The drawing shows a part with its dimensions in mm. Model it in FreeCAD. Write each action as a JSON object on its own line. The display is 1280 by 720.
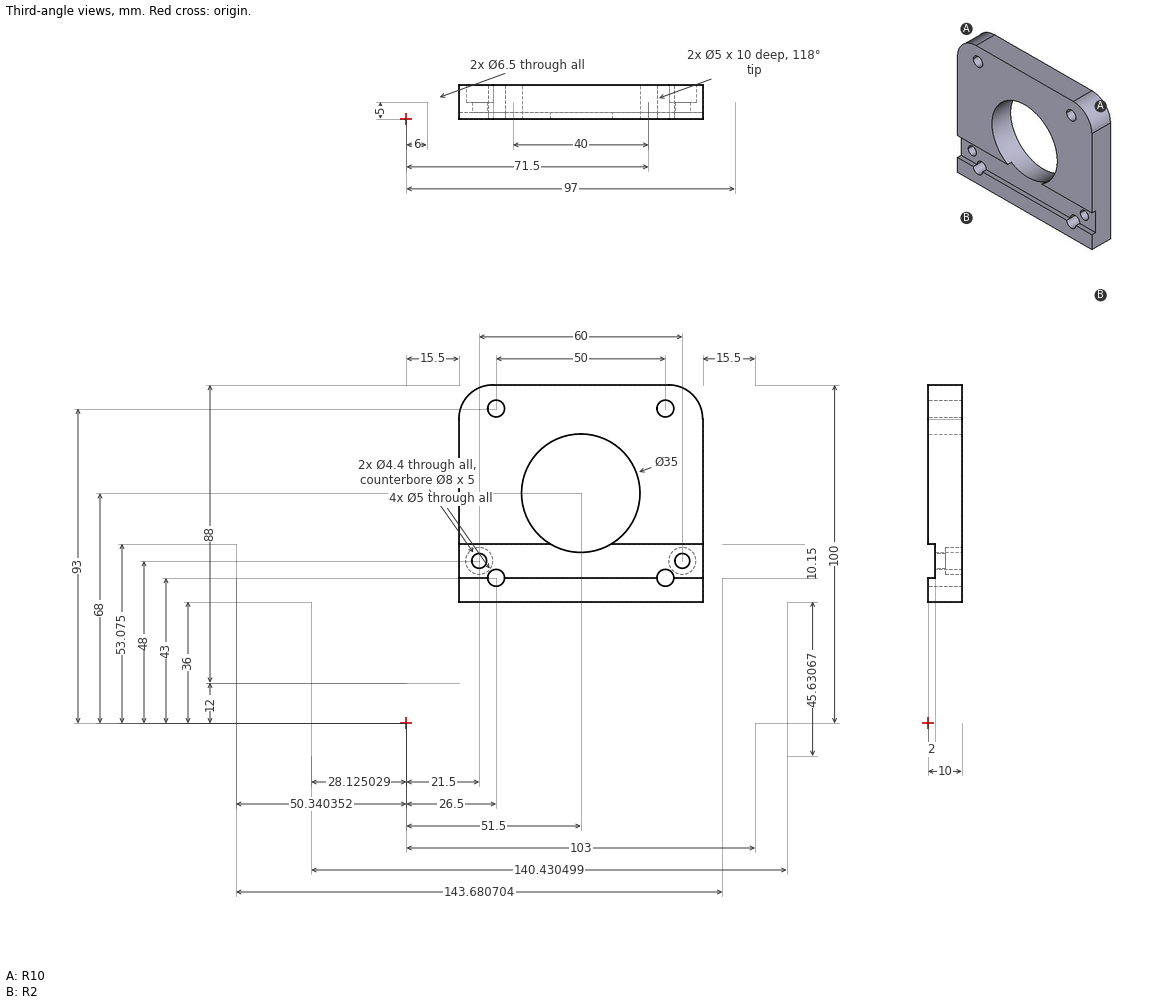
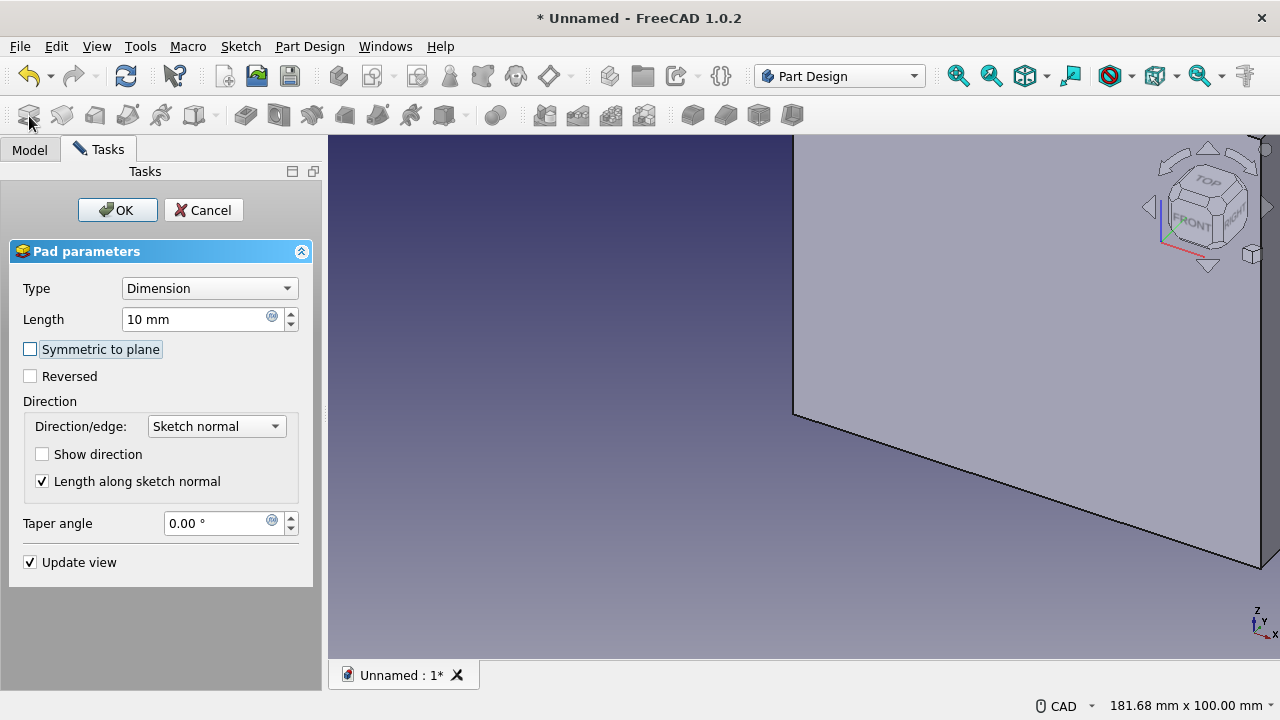
{"action": "left_click", "coordinate": [31, 376]}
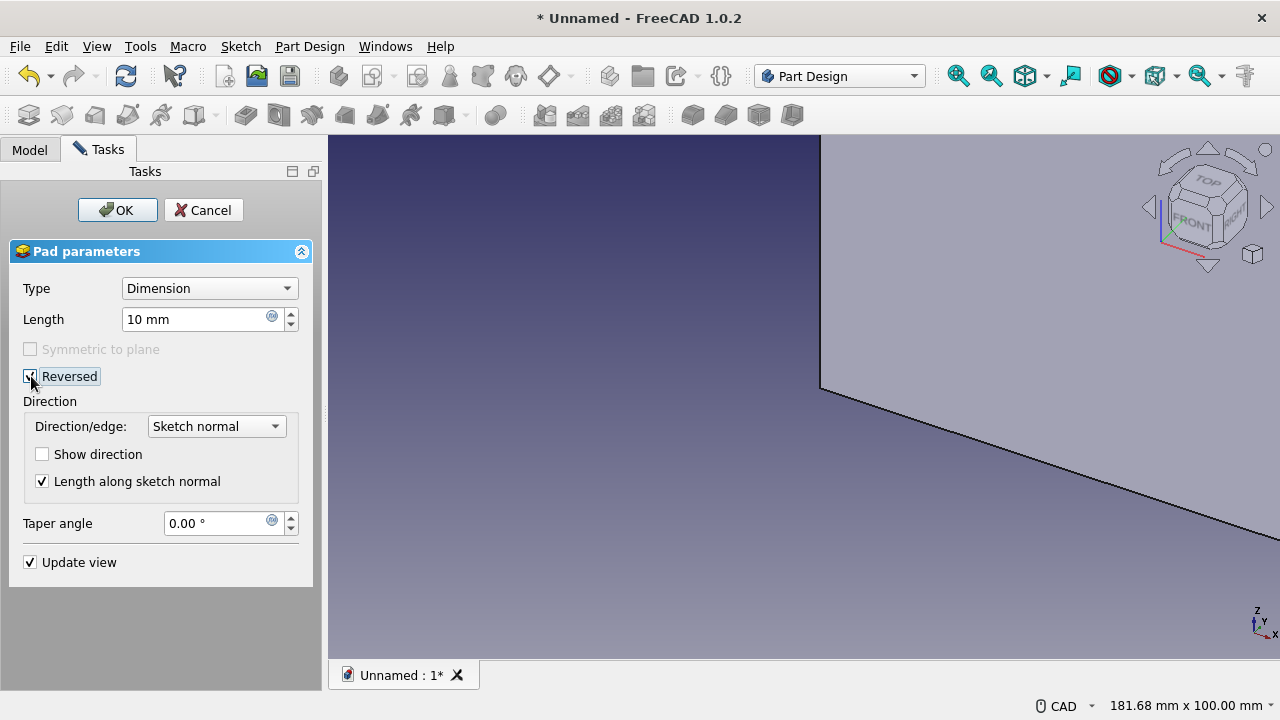
{"action": "left_click", "coordinate": [118, 210]}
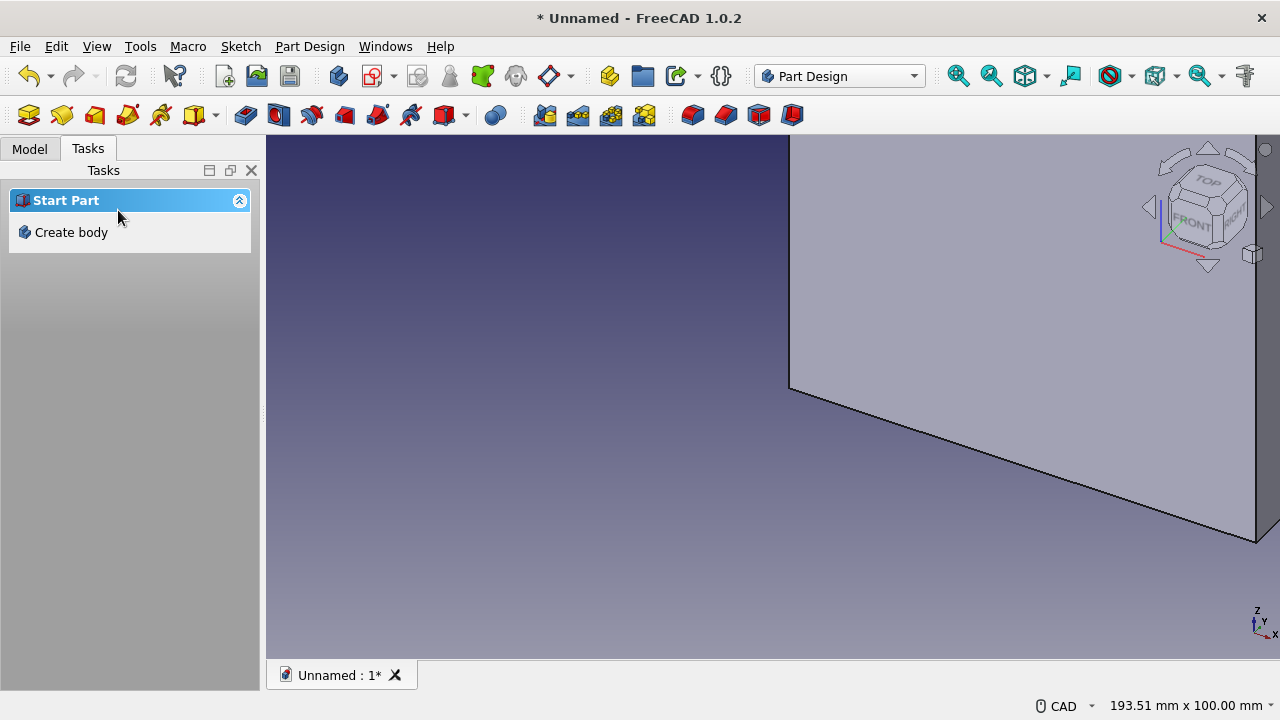
{"action": "left_click", "coordinate": [959, 76]}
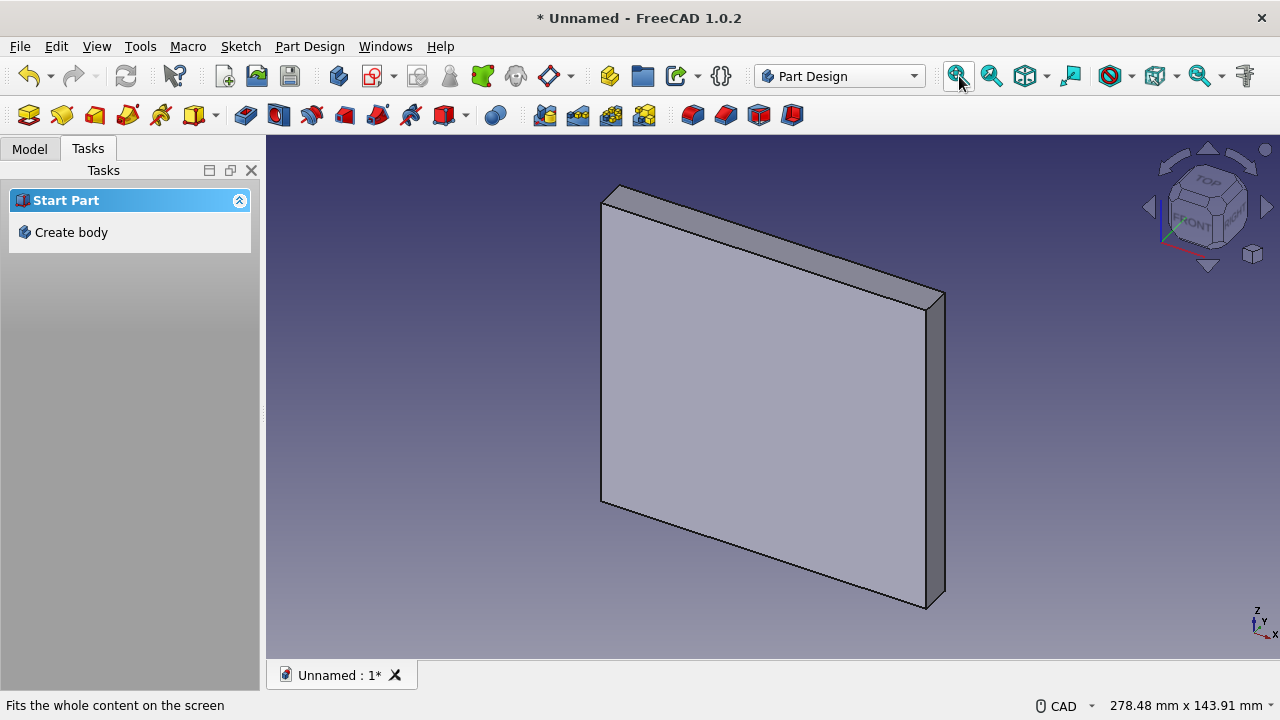
{"action": "key", "text": "4"}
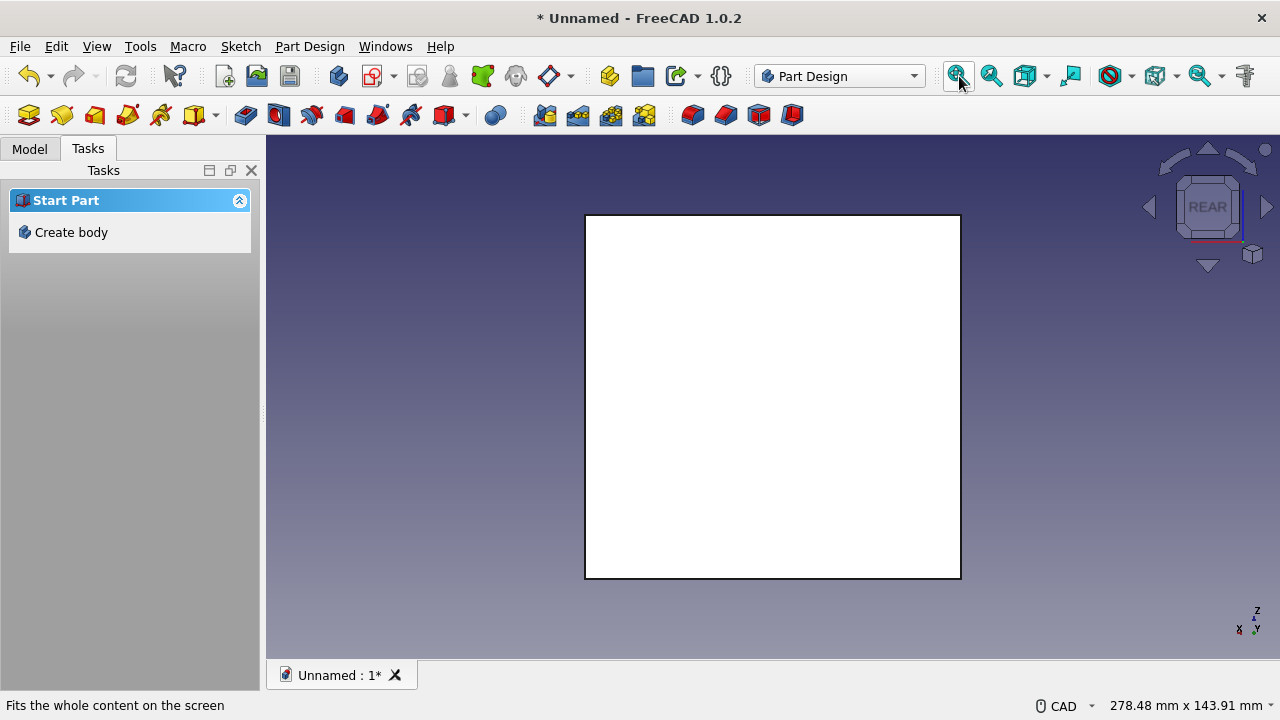
{"action": "left_click", "coordinate": [773, 396]}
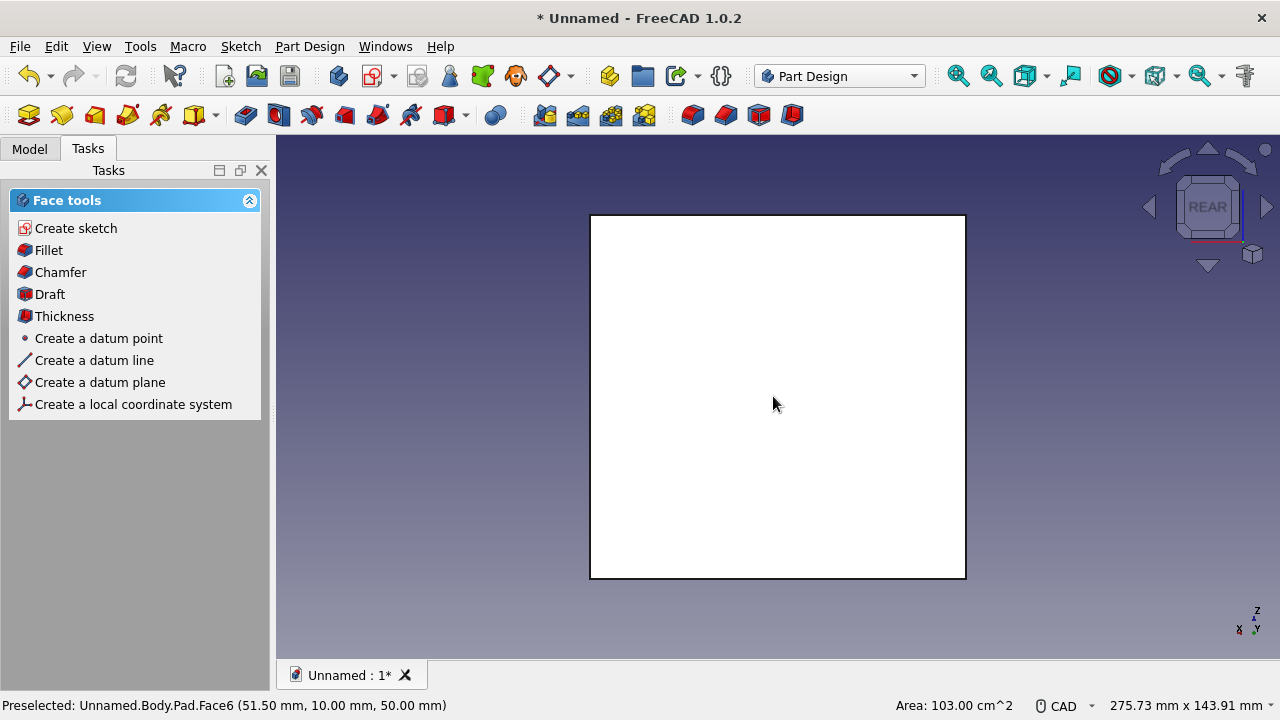
{"action": "left_click", "coordinate": [372, 76]}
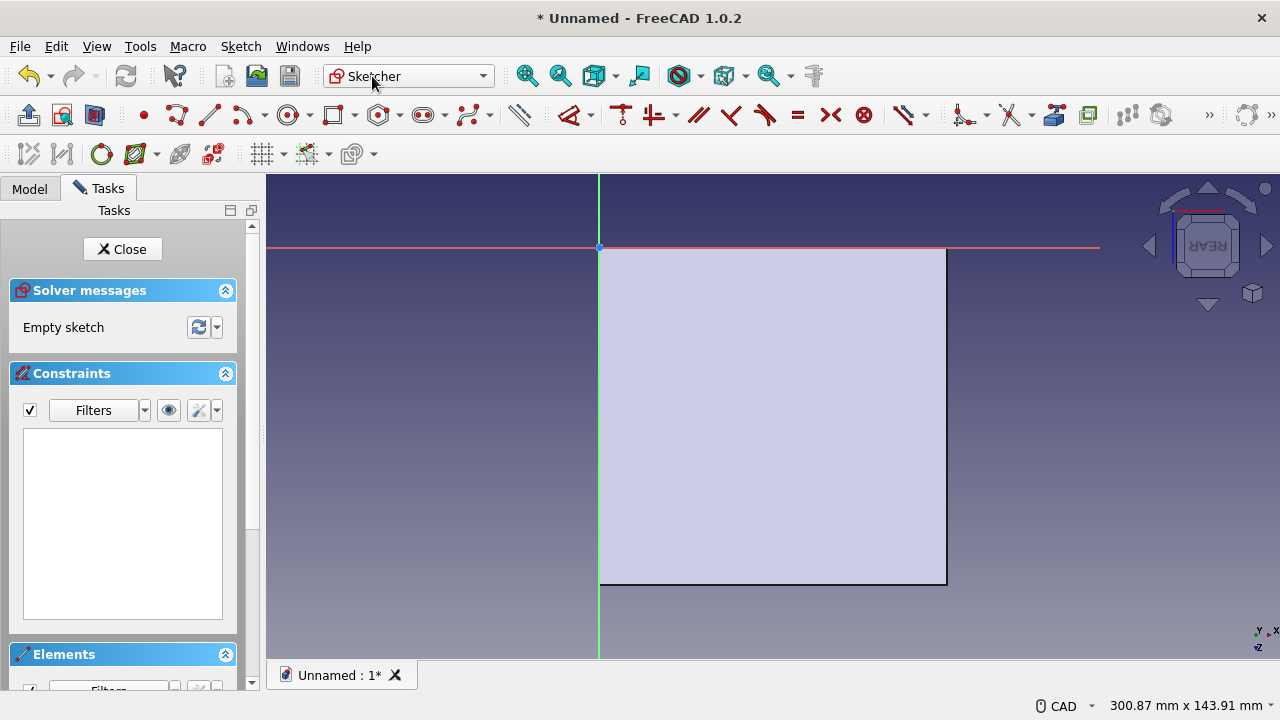
{"action": "left_click", "coordinate": [332, 116]}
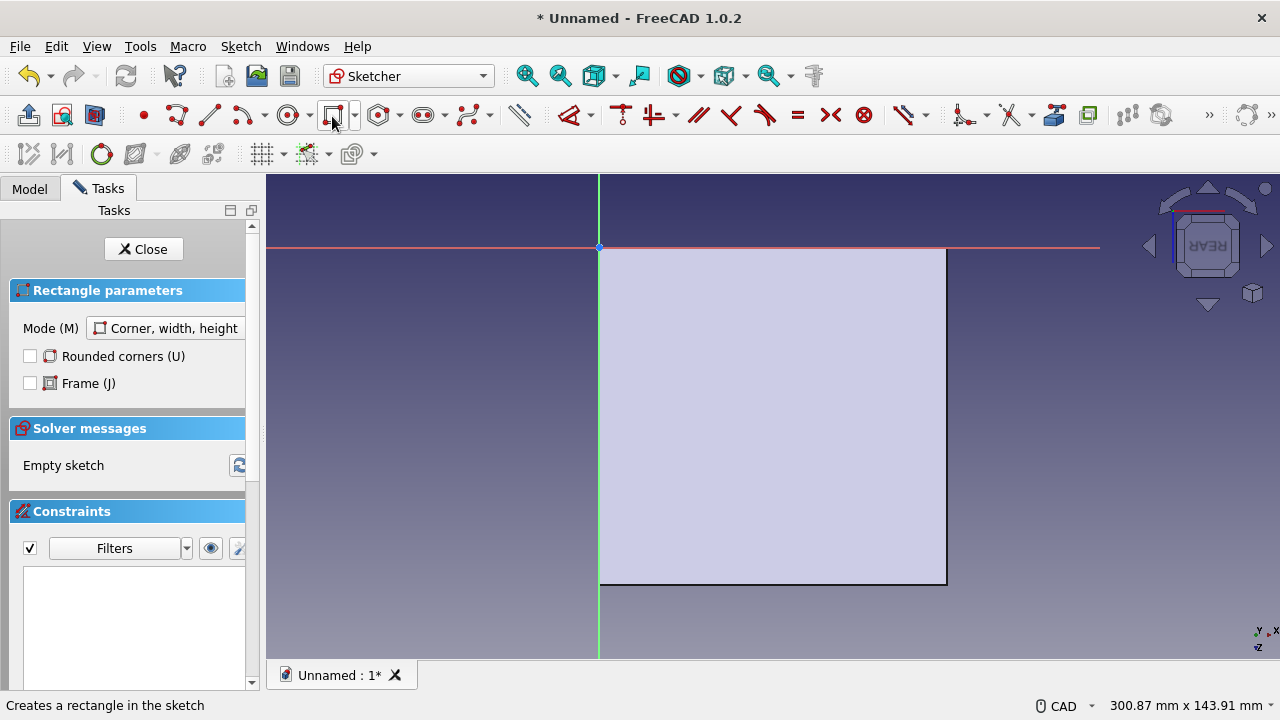
{"action": "left_click", "coordinate": [599, 288]}
{"action": "mouse_move", "coordinate": [652, 585]}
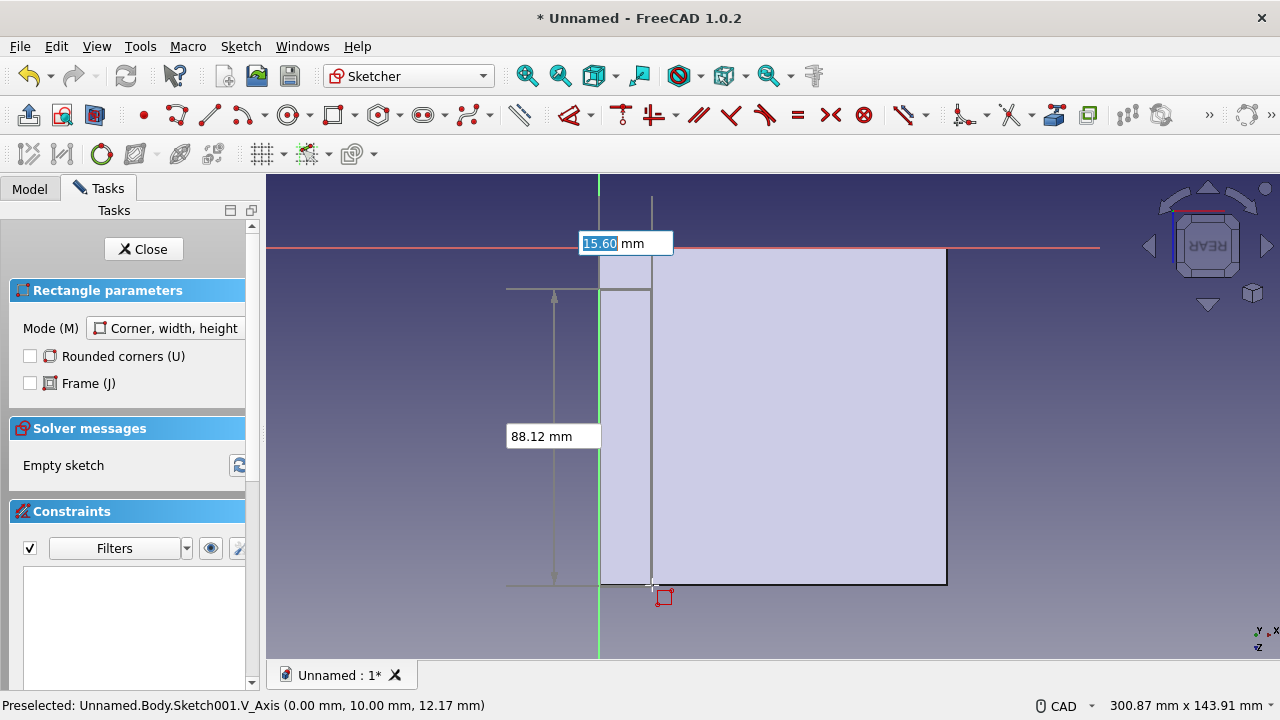
{"action": "type", "text": "15.5"}
{"action": "key", "text": "Tab"}
{"action": "type", "text": "88"}
{"action": "key", "text": "Return"}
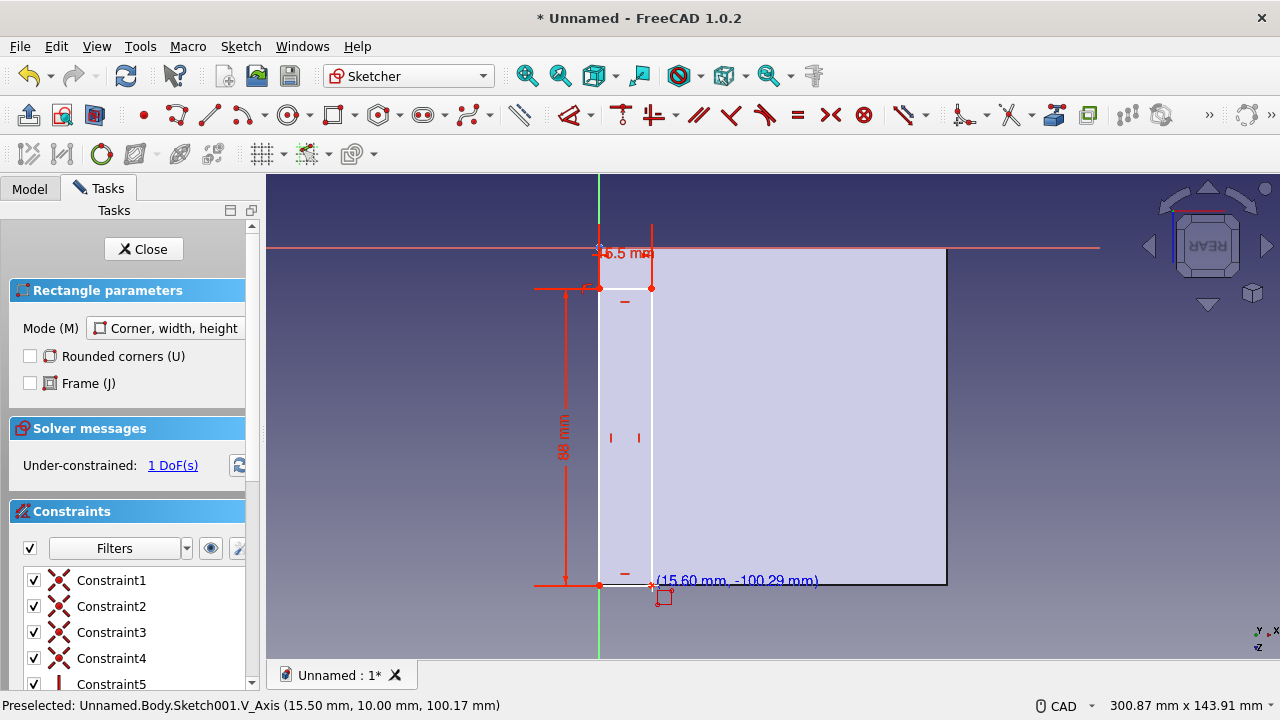
{"action": "left_click", "coordinate": [894, 288]}
{"action": "mouse_move", "coordinate": [947, 585]}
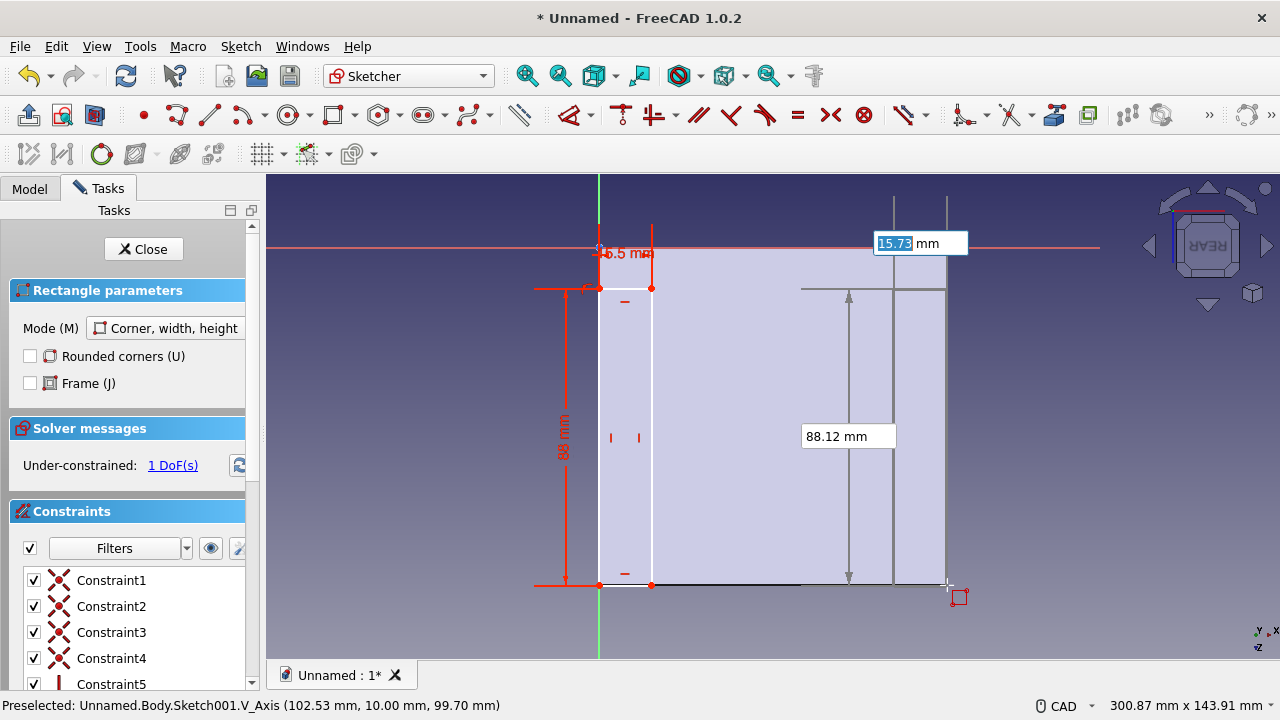
{"action": "type", "text": "15.5"}
{"action": "key", "text": "Tab"}
{"action": "type", "text": "88"}
{"action": "key", "text": "Return"}
{"action": "key", "text": "Escape"}